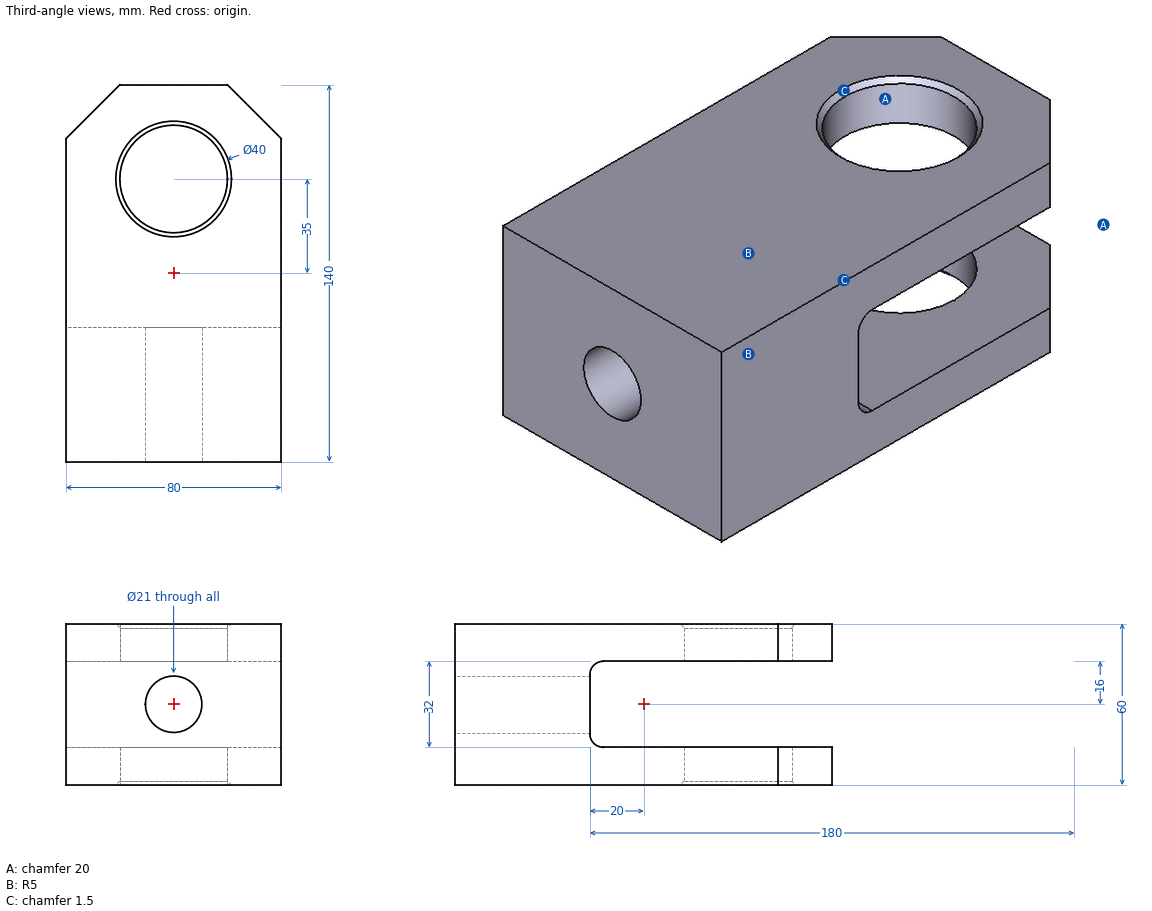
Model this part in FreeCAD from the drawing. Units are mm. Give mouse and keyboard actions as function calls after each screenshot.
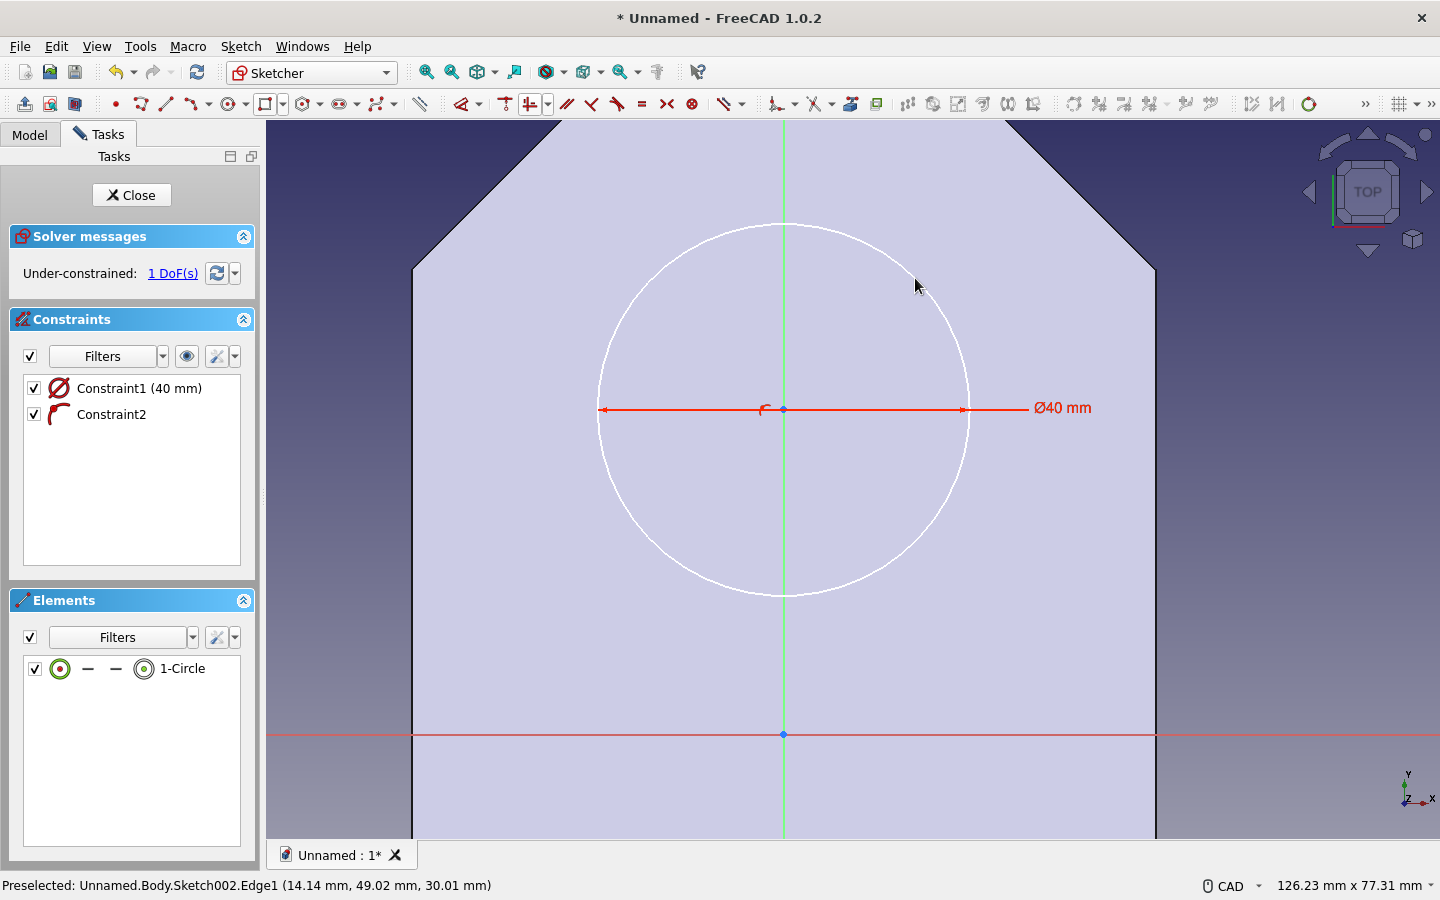
click(460, 104)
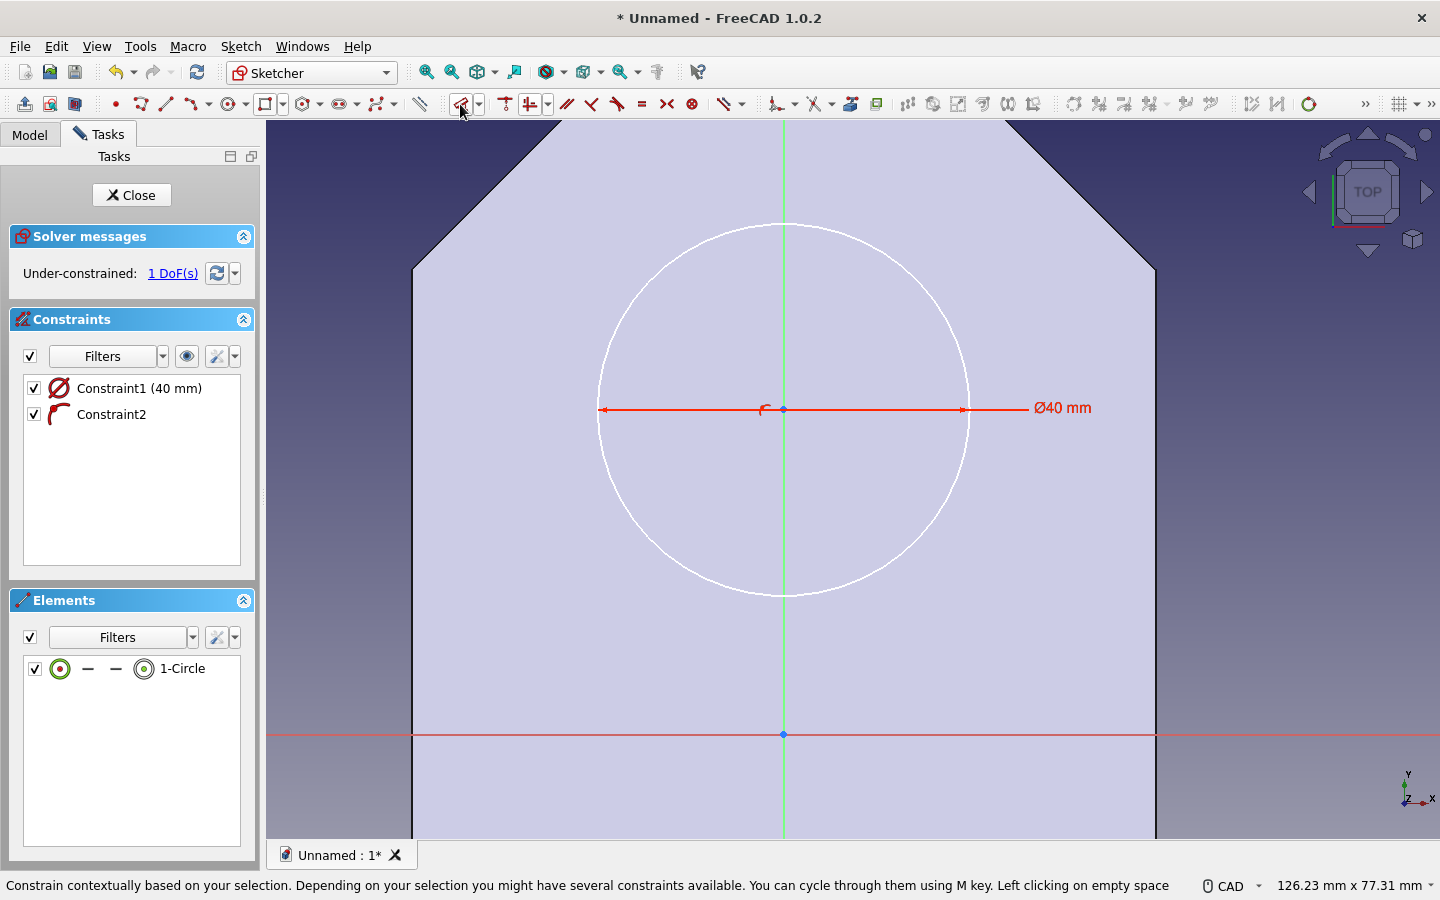
click(784, 410)
click(818, 572)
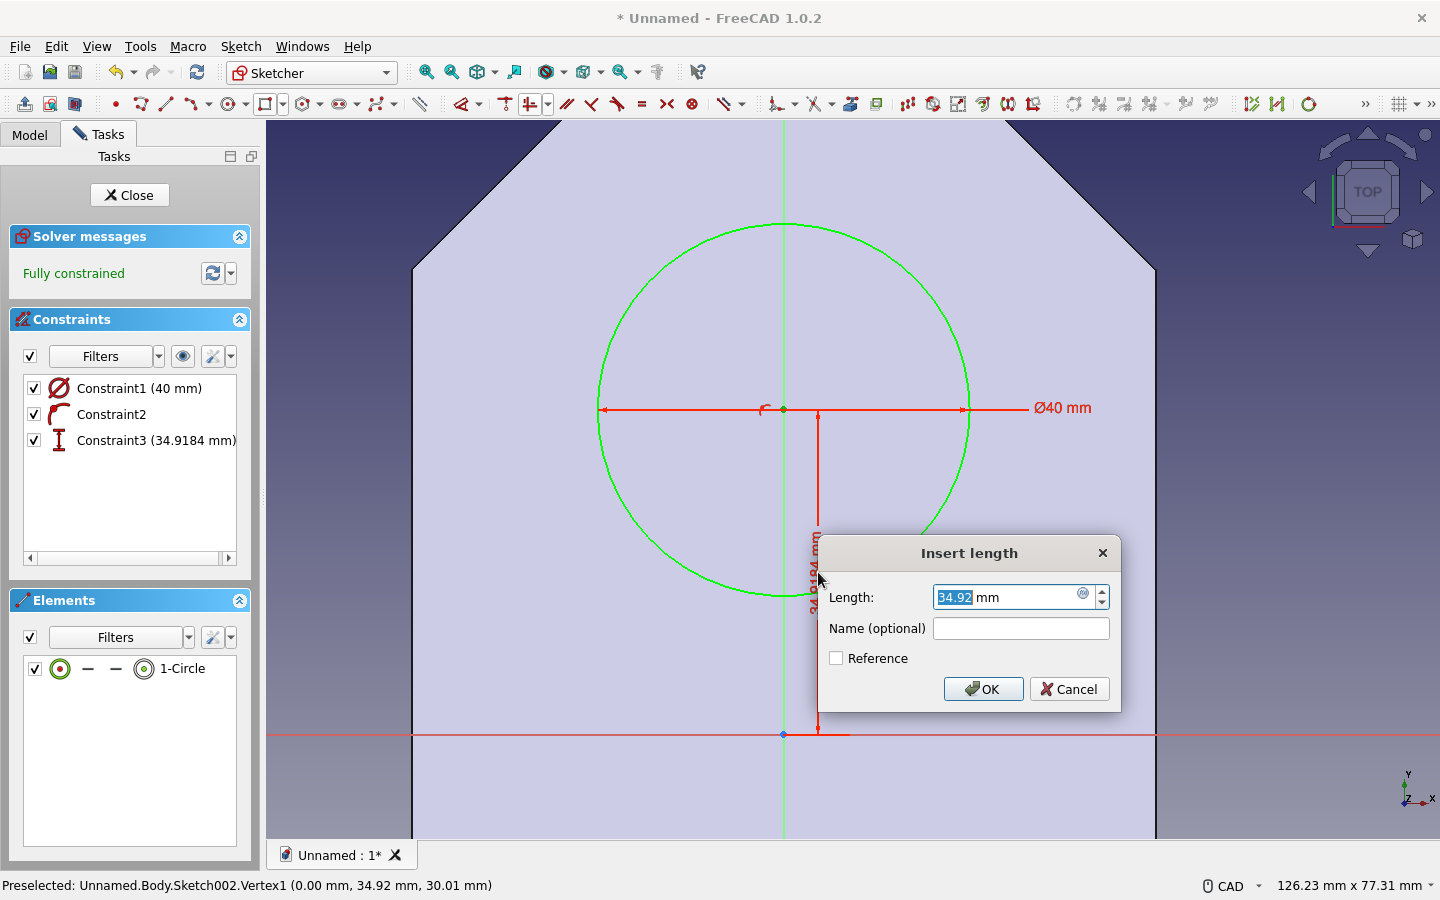
text(35)
key(Return)
key(Escape)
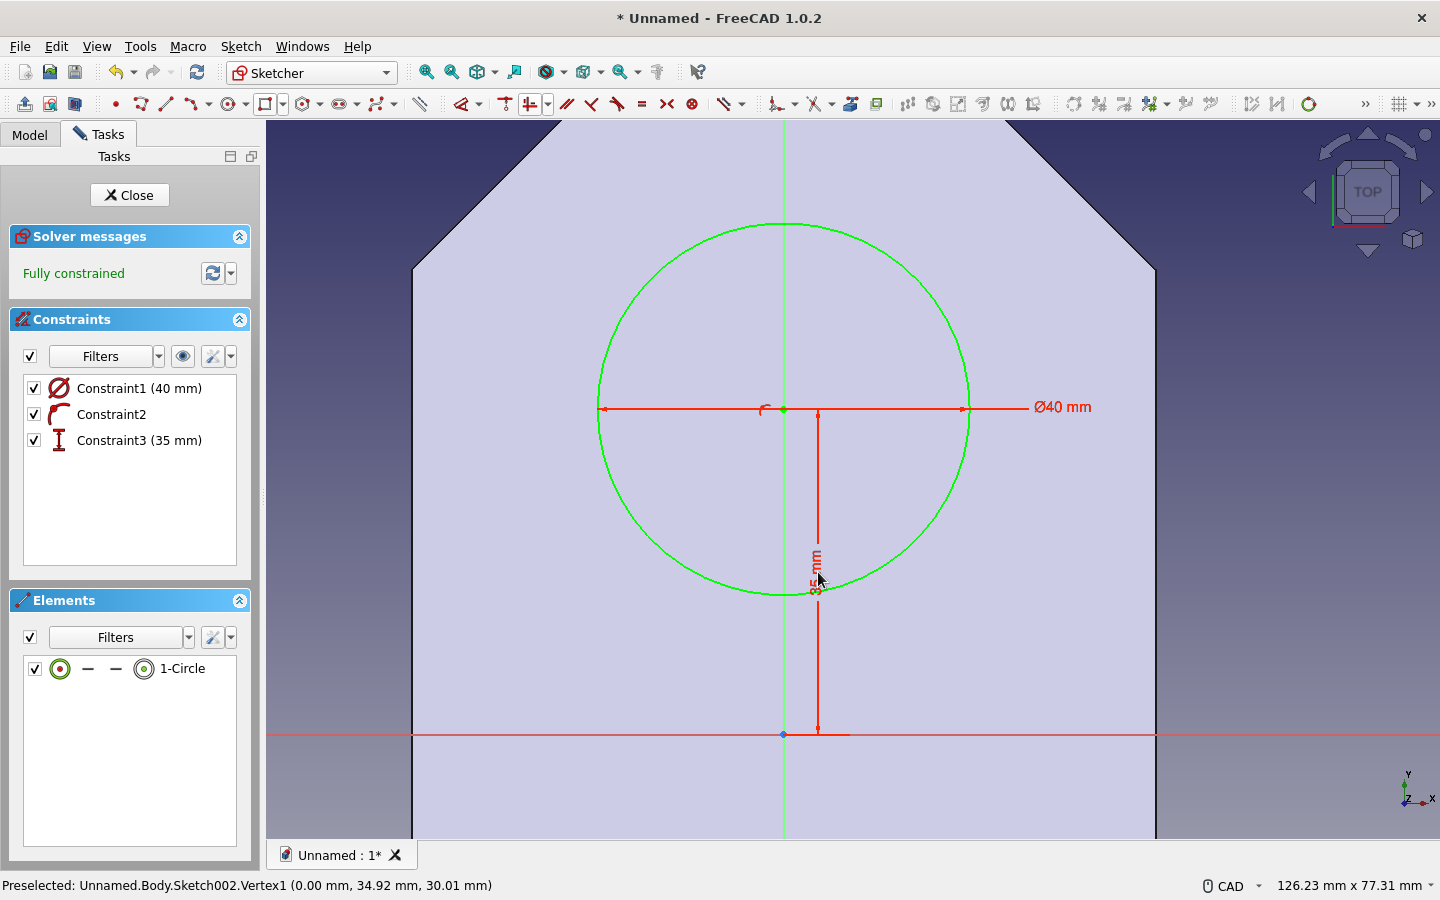
click(130, 195)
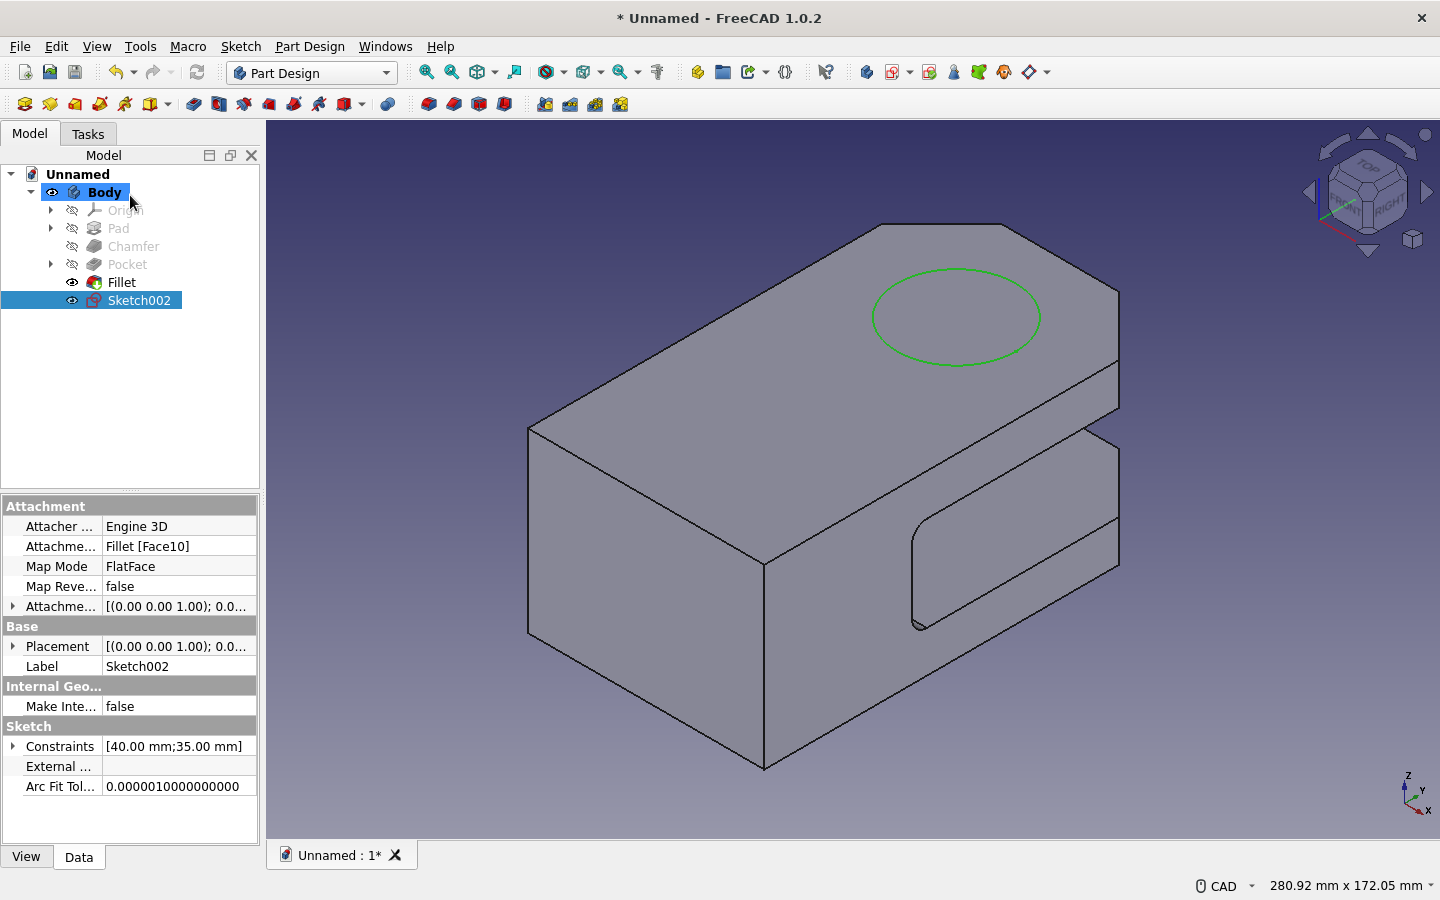
click(194, 104)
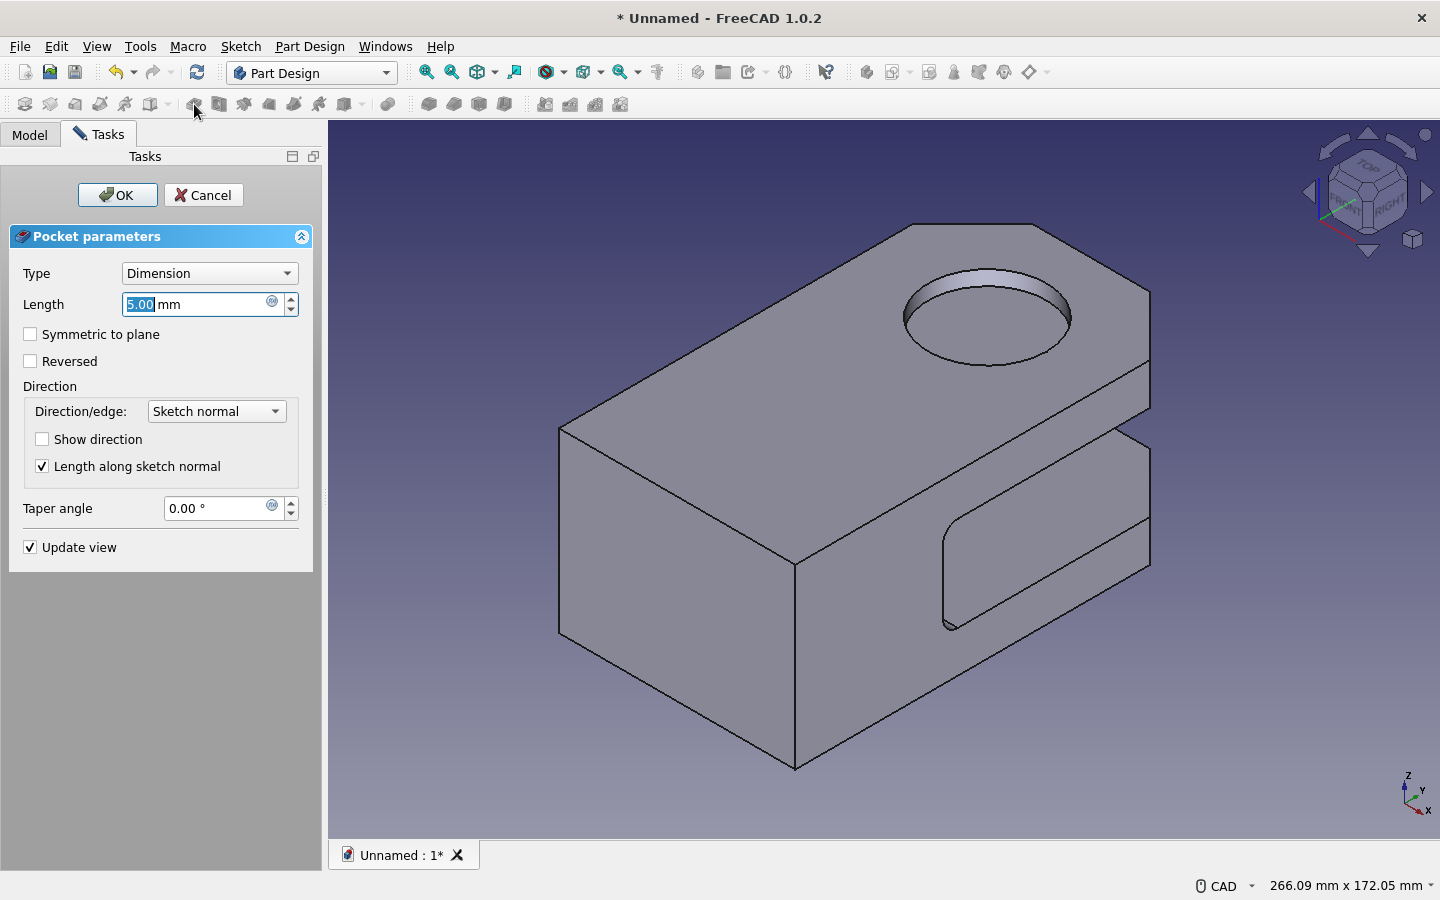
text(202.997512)
key(Tab)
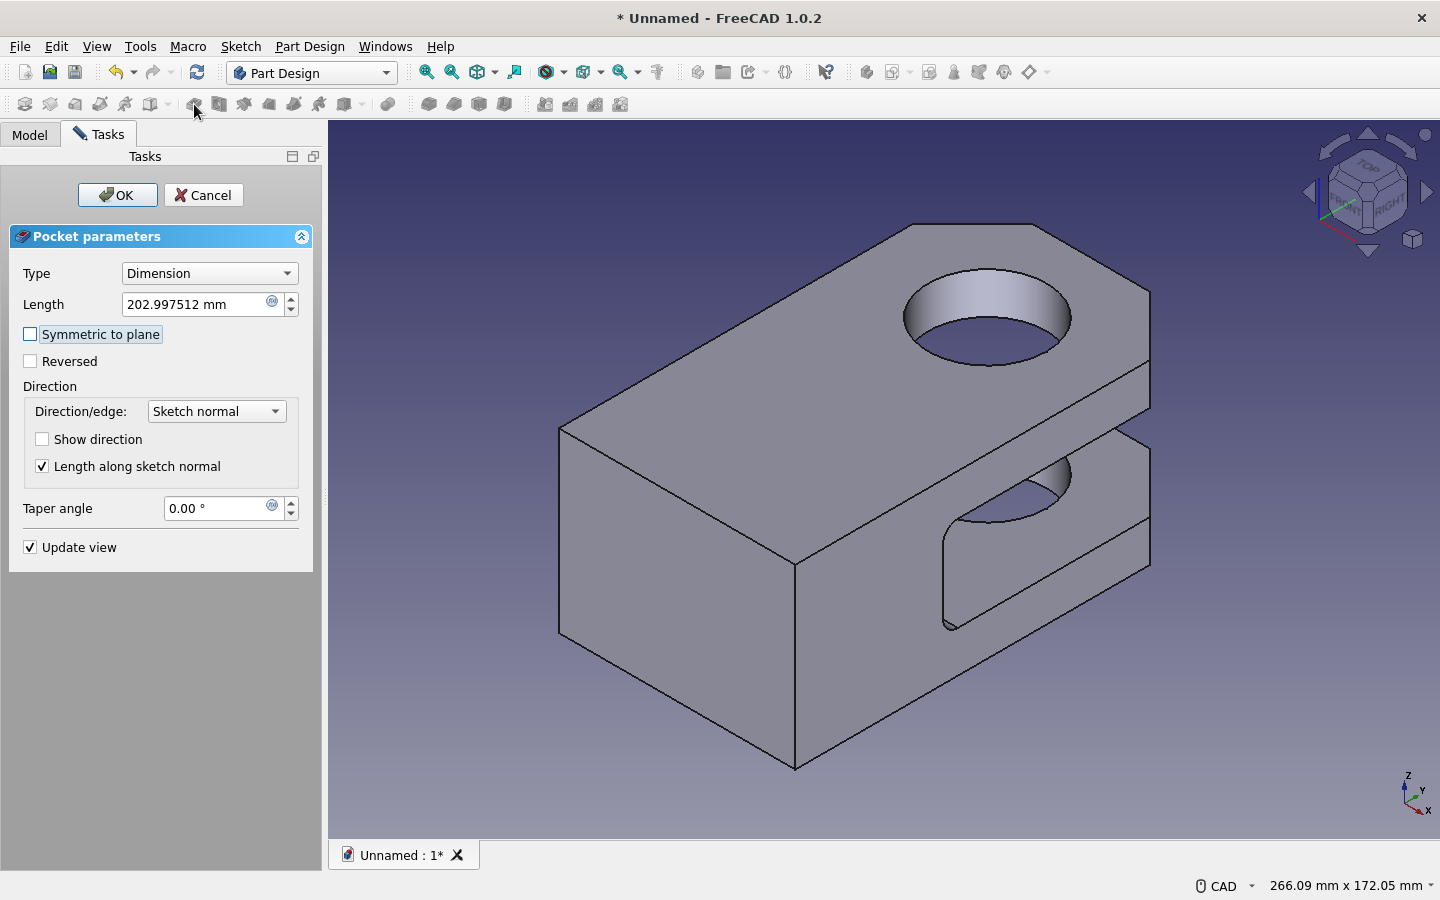
click(31, 334)